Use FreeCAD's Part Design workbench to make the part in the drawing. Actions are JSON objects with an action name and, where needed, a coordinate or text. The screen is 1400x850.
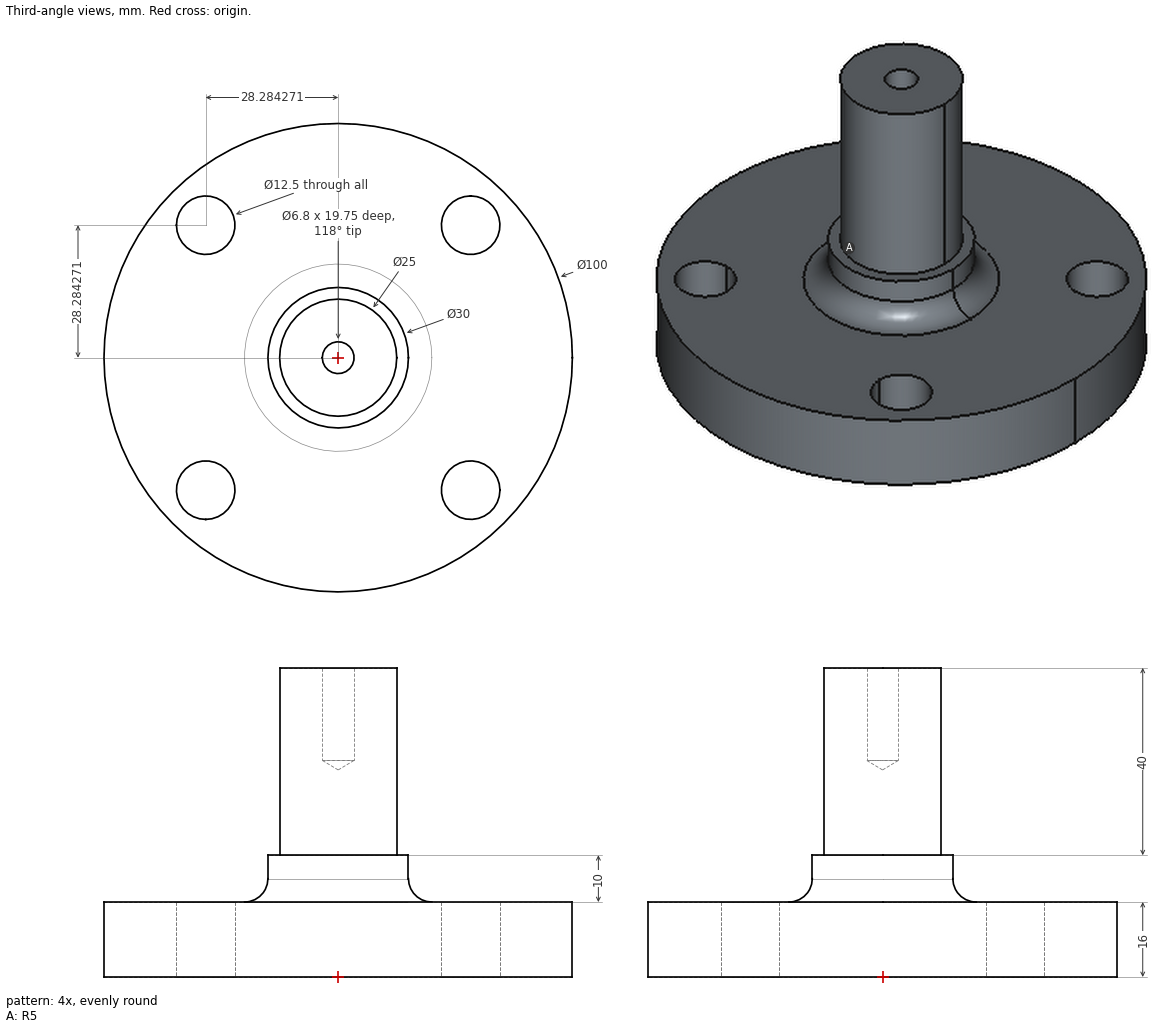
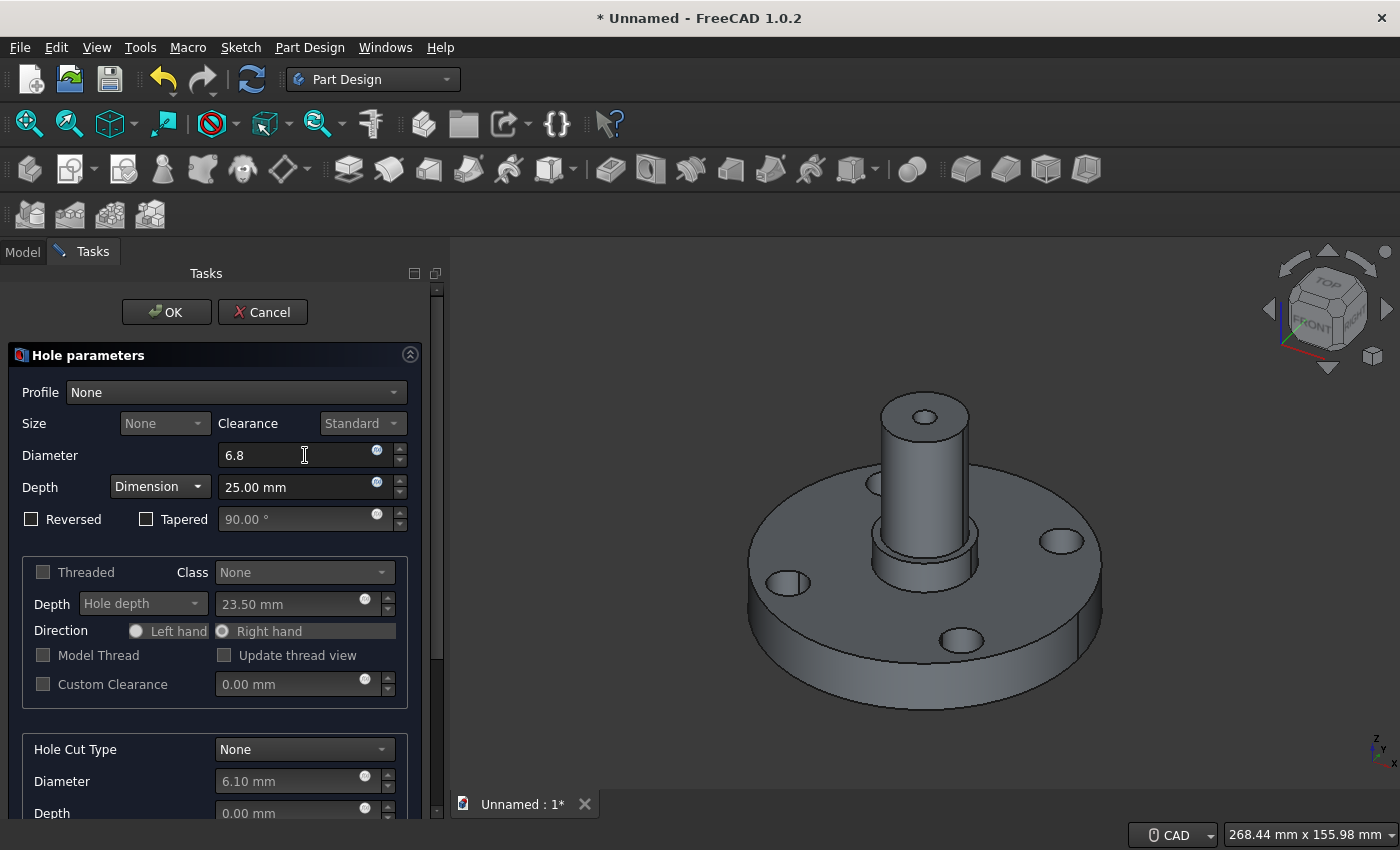
{"action": "triple_click", "coordinate": [305, 487]}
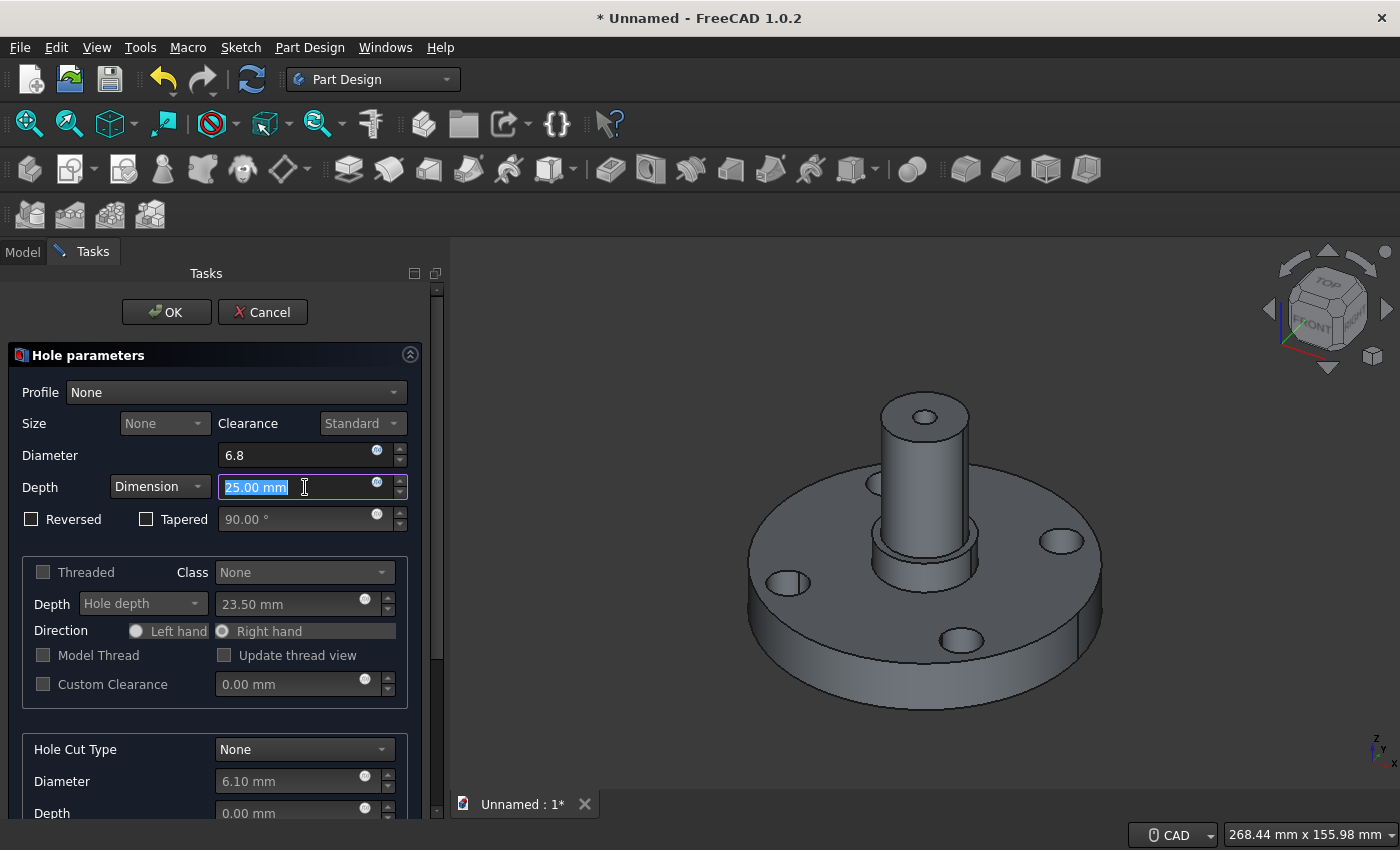
{"action": "type", "text": "19.75"}
{"action": "key", "text": "Tab"}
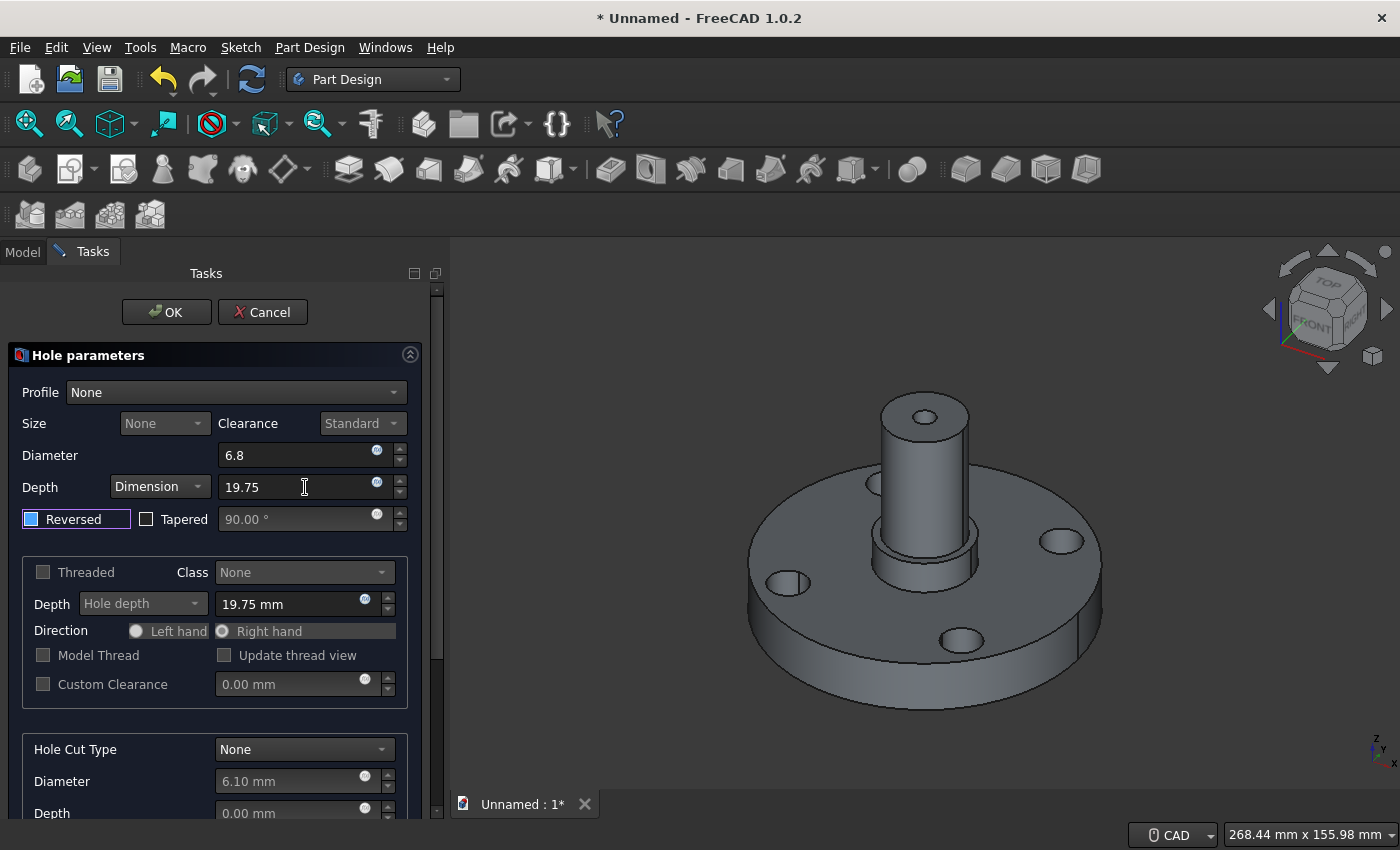
{"action": "left_click", "coordinate": [167, 312]}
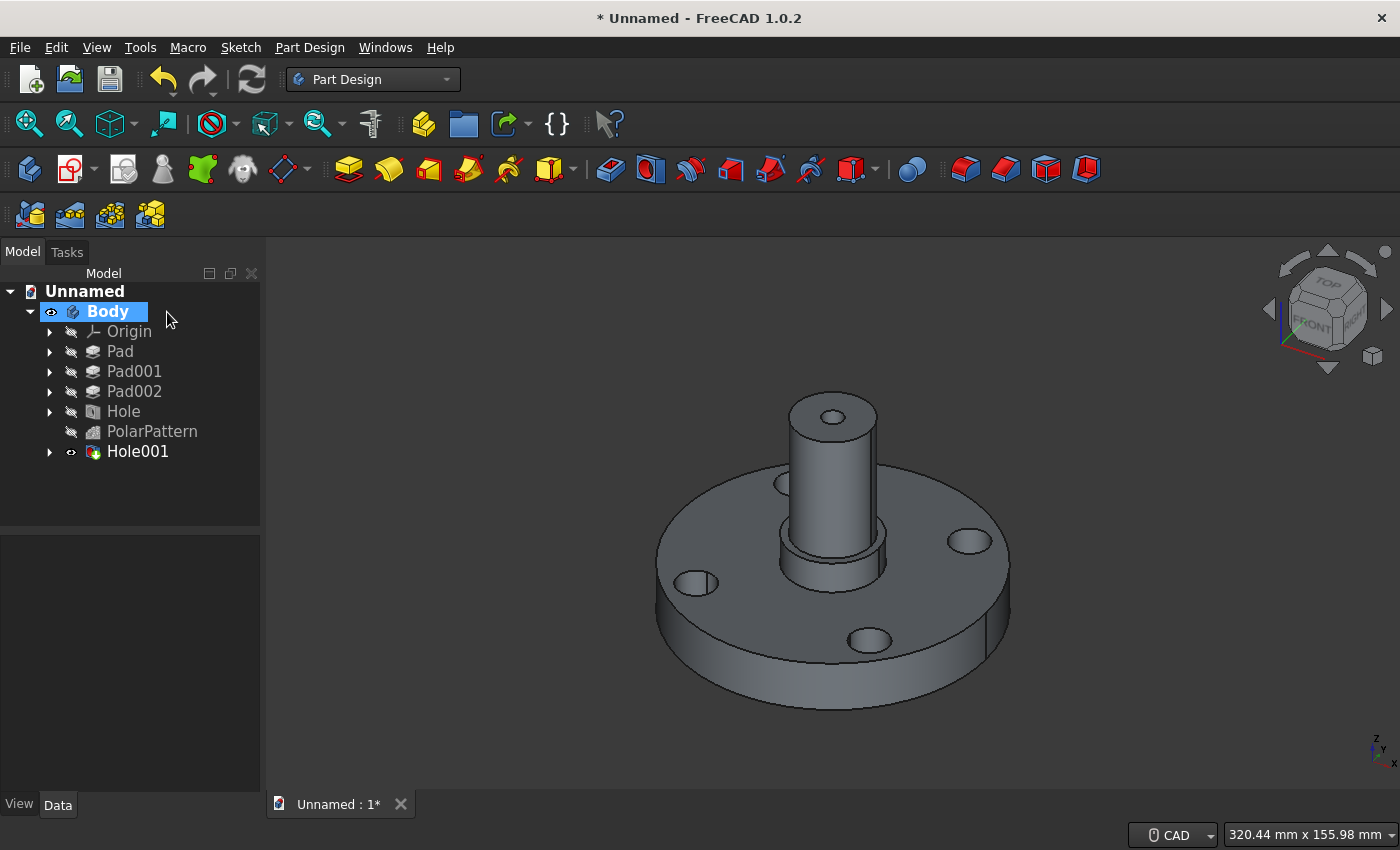
{"action": "key", "text": "0"}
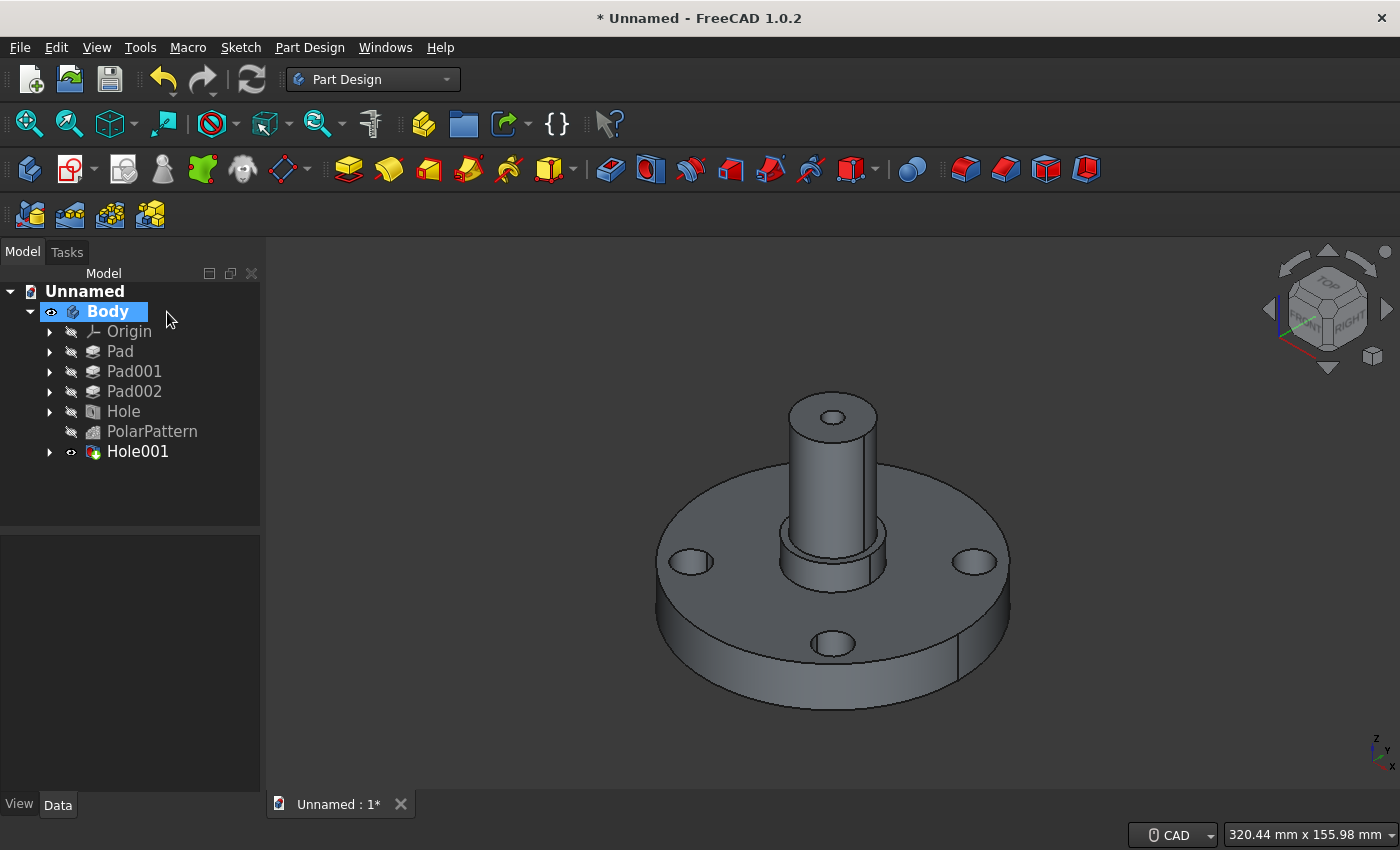
{"action": "key", "text": "2"}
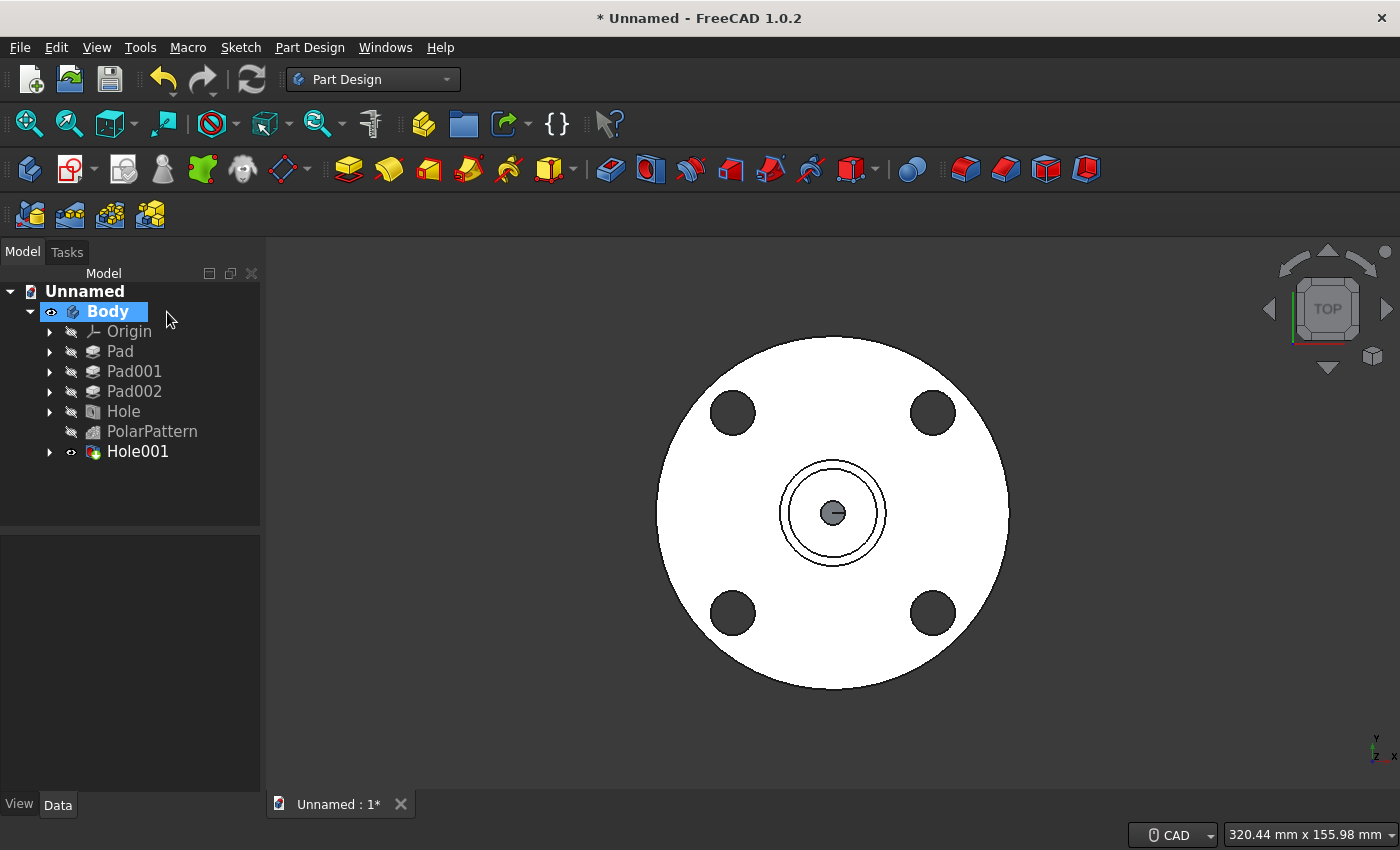
{"action": "key", "text": "1"}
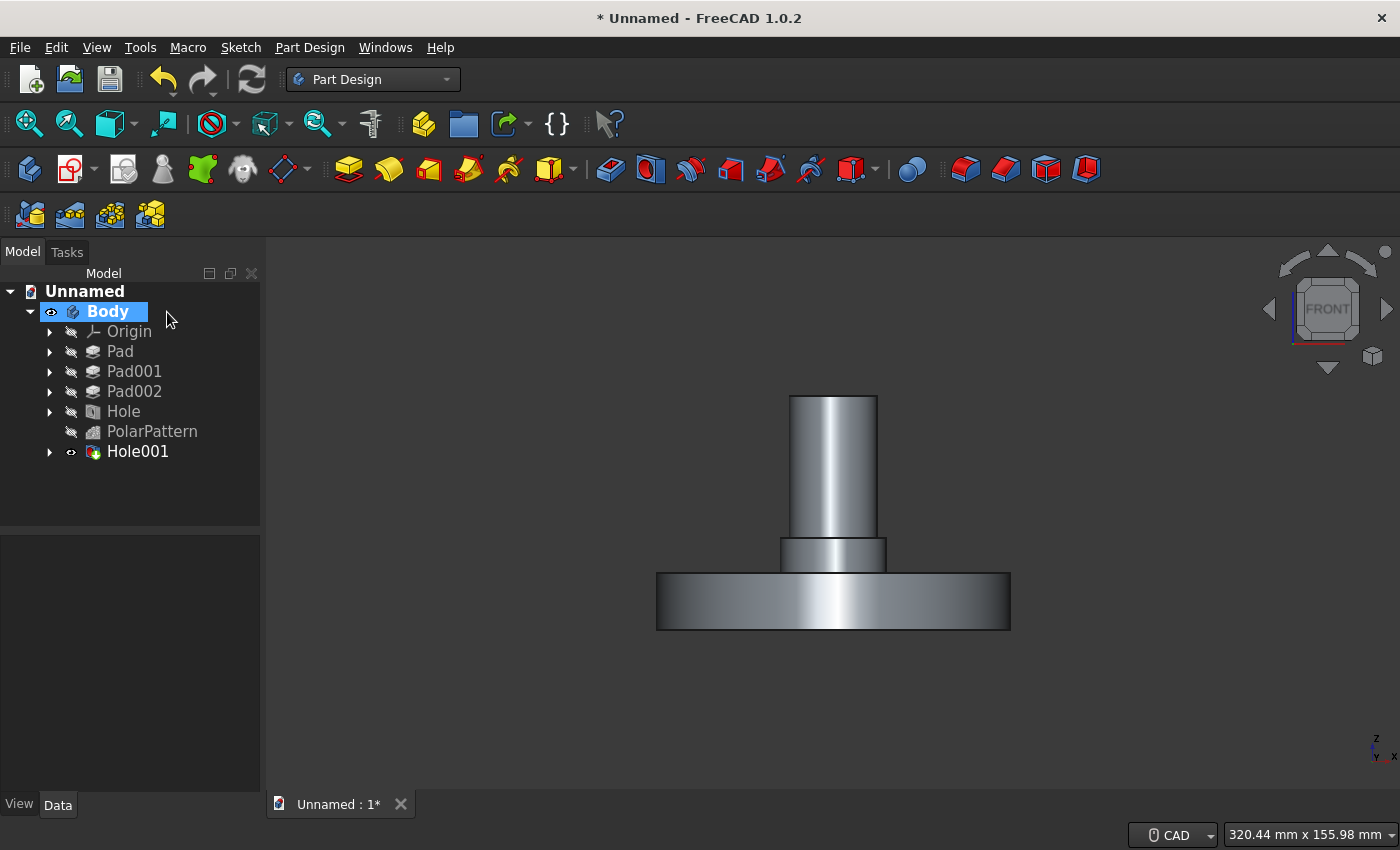
{"action": "left_click", "coordinate": [30, 124]}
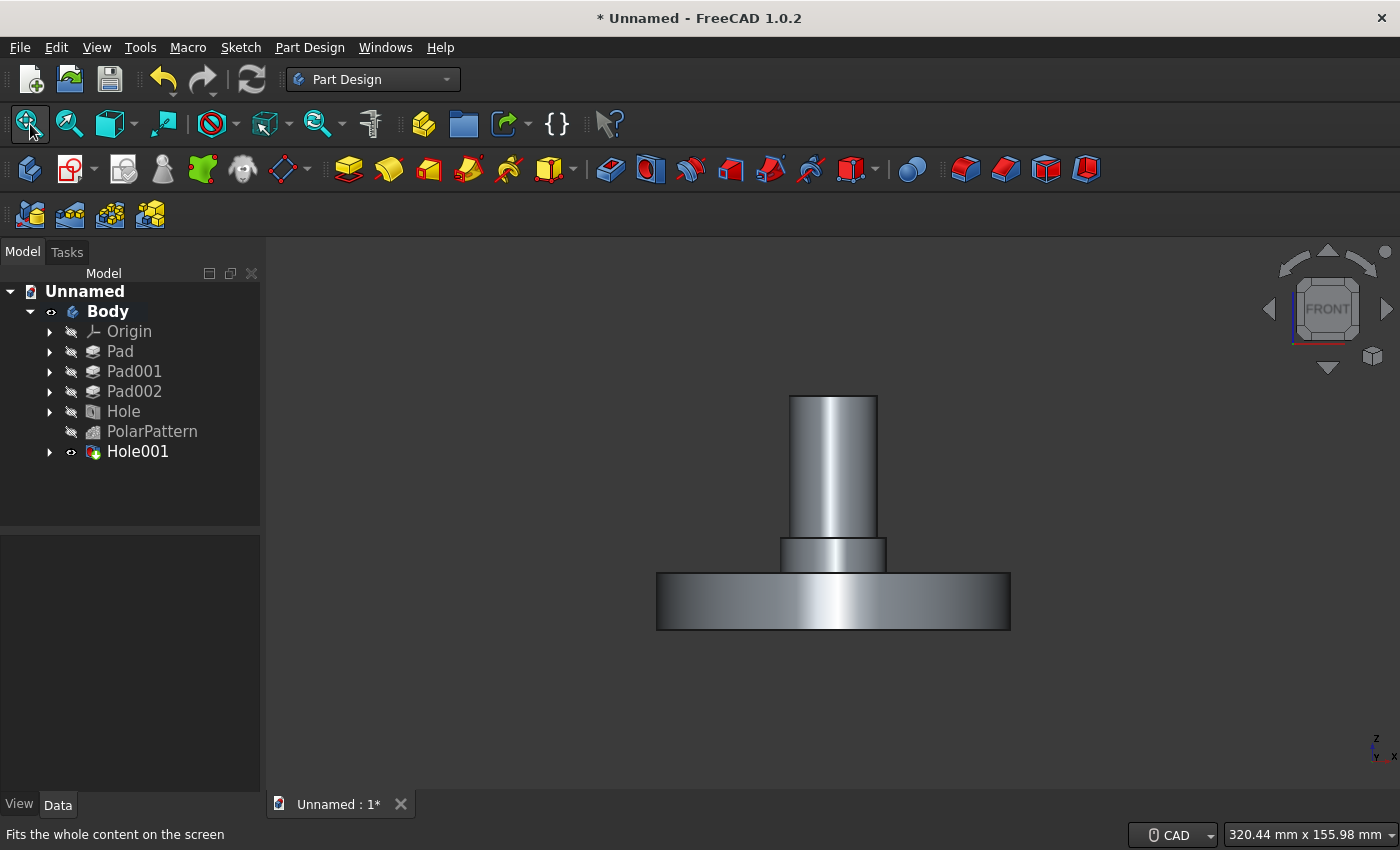
{"action": "key", "text": "3"}